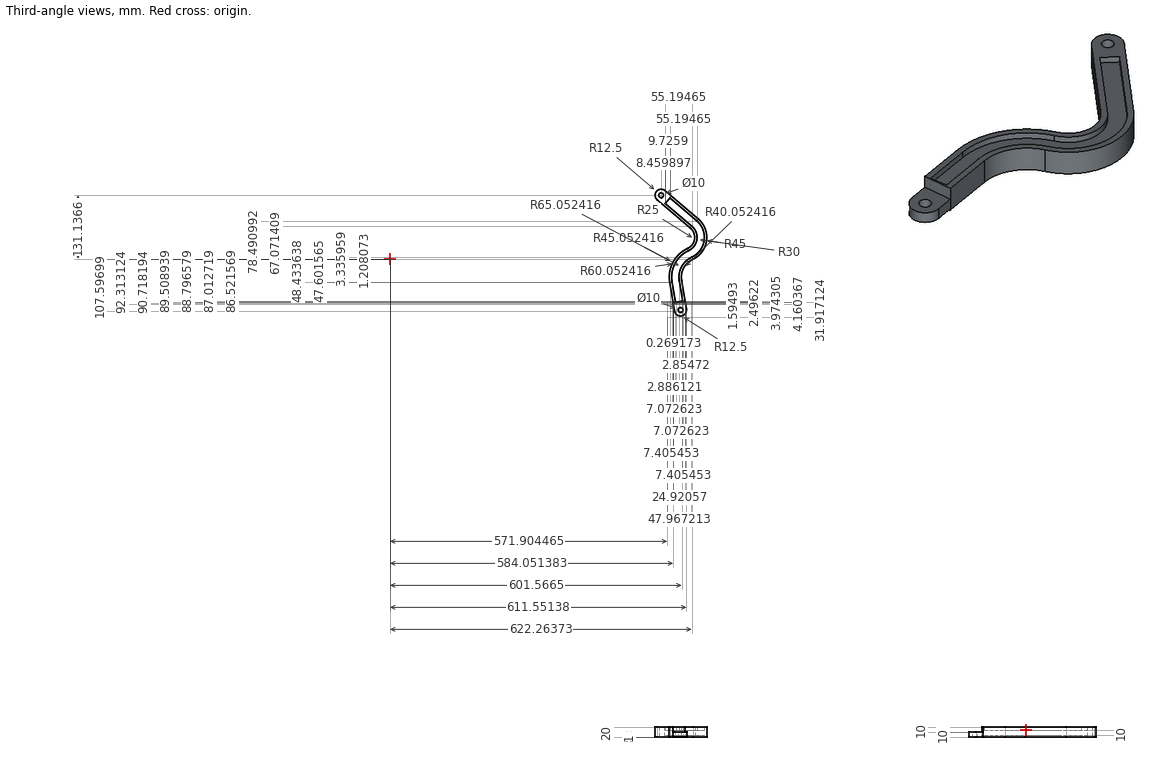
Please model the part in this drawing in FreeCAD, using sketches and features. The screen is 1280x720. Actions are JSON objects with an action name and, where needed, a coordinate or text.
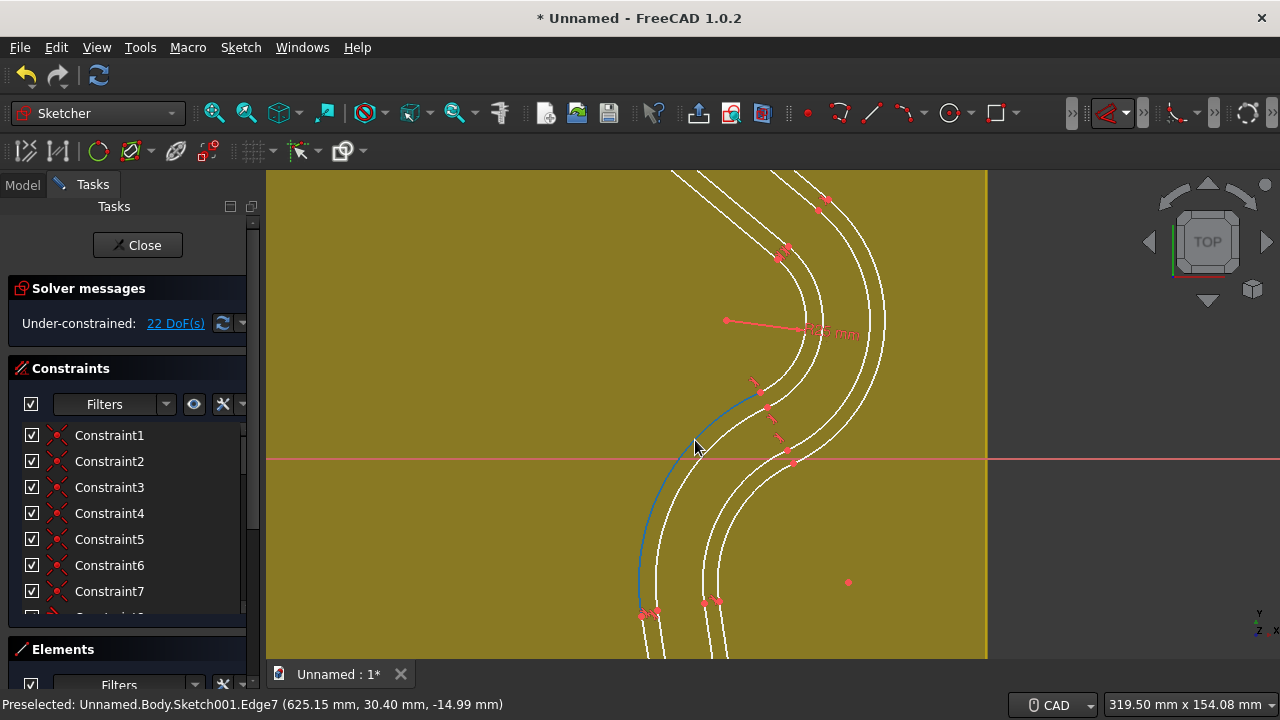
{"action": "left_click", "coordinate": [695, 440]}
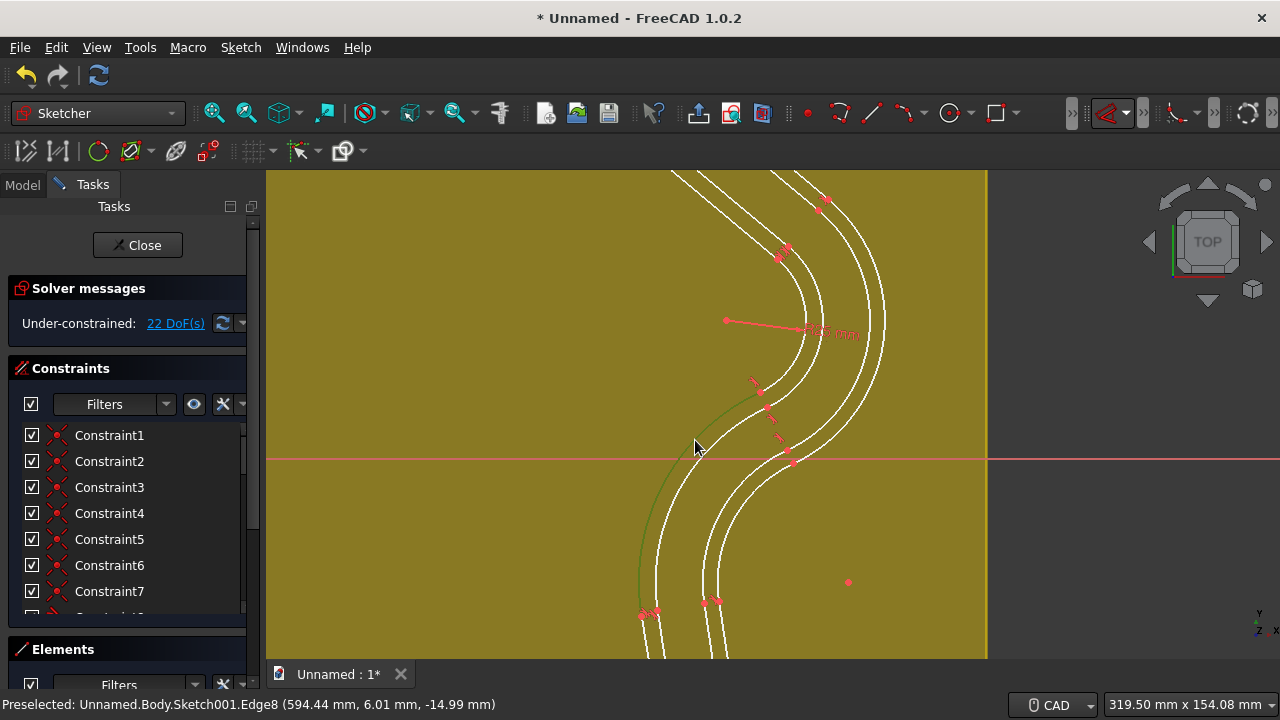
{"action": "key", "text": "k r"}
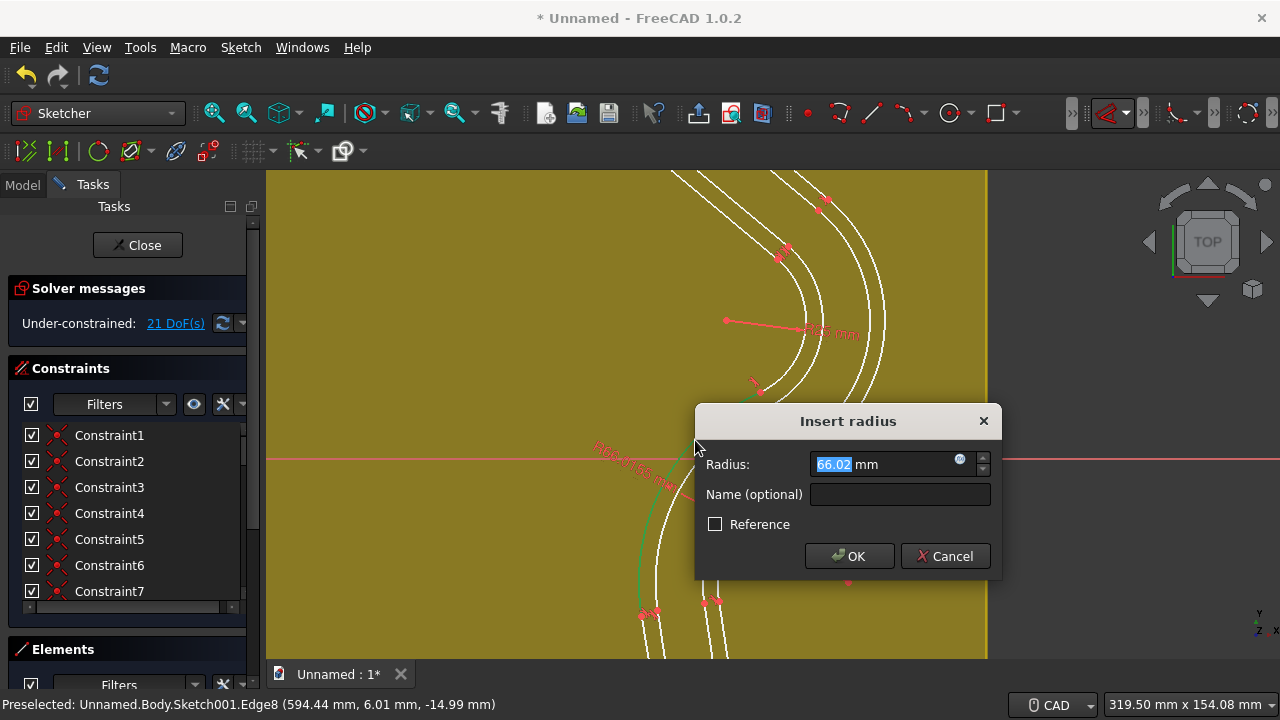
{"action": "type", "text": "65.052416"}
{"action": "key", "text": "Return"}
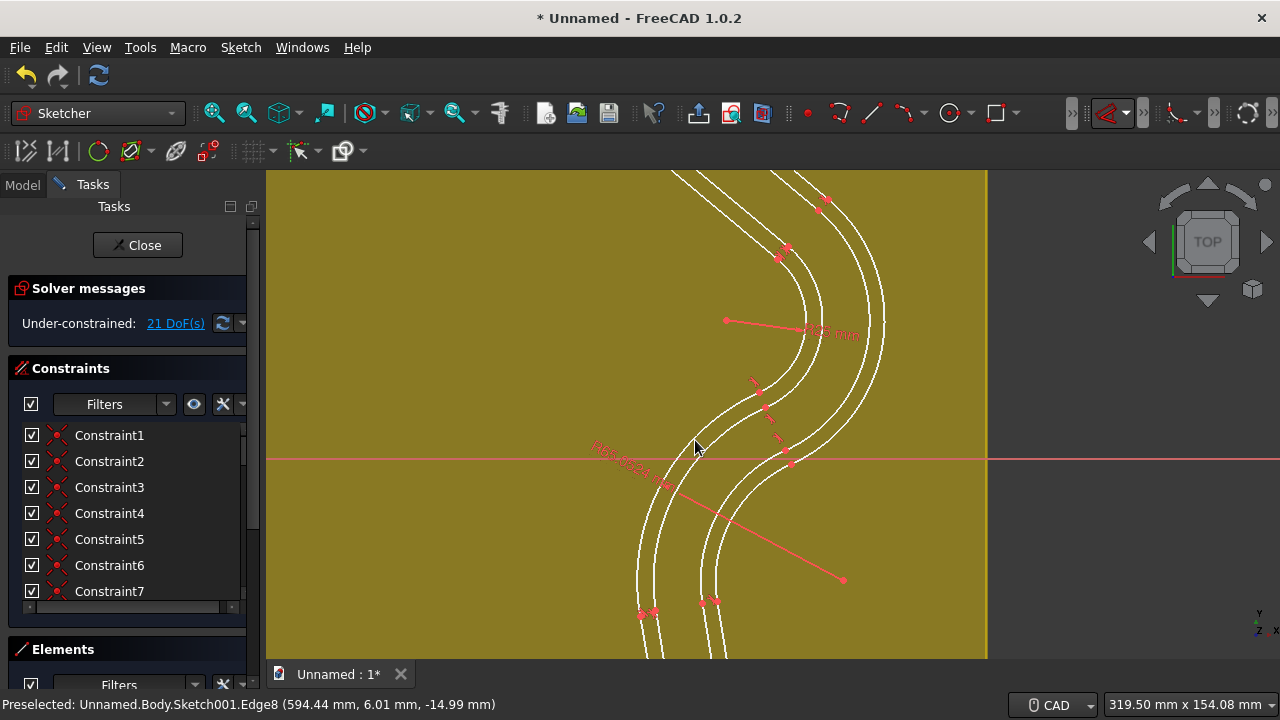
{"action": "left_click", "coordinate": [751, 493]}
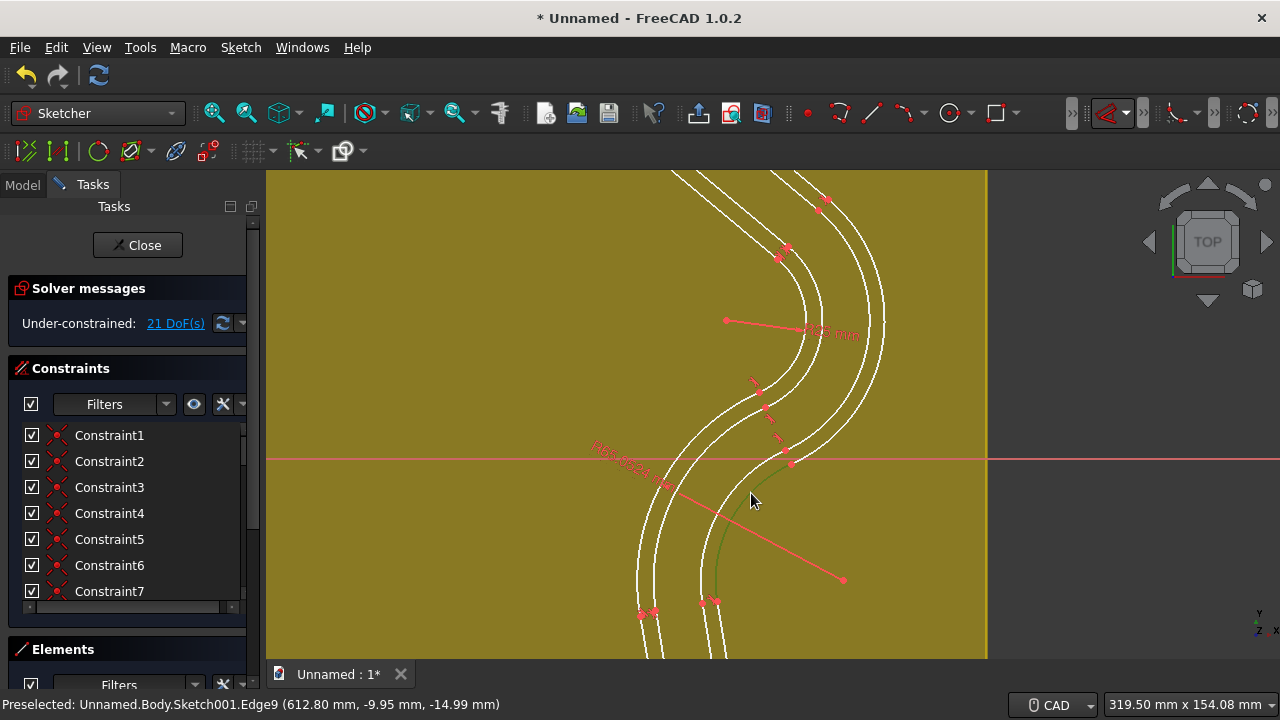
{"action": "left_click", "coordinate": [1128, 114]}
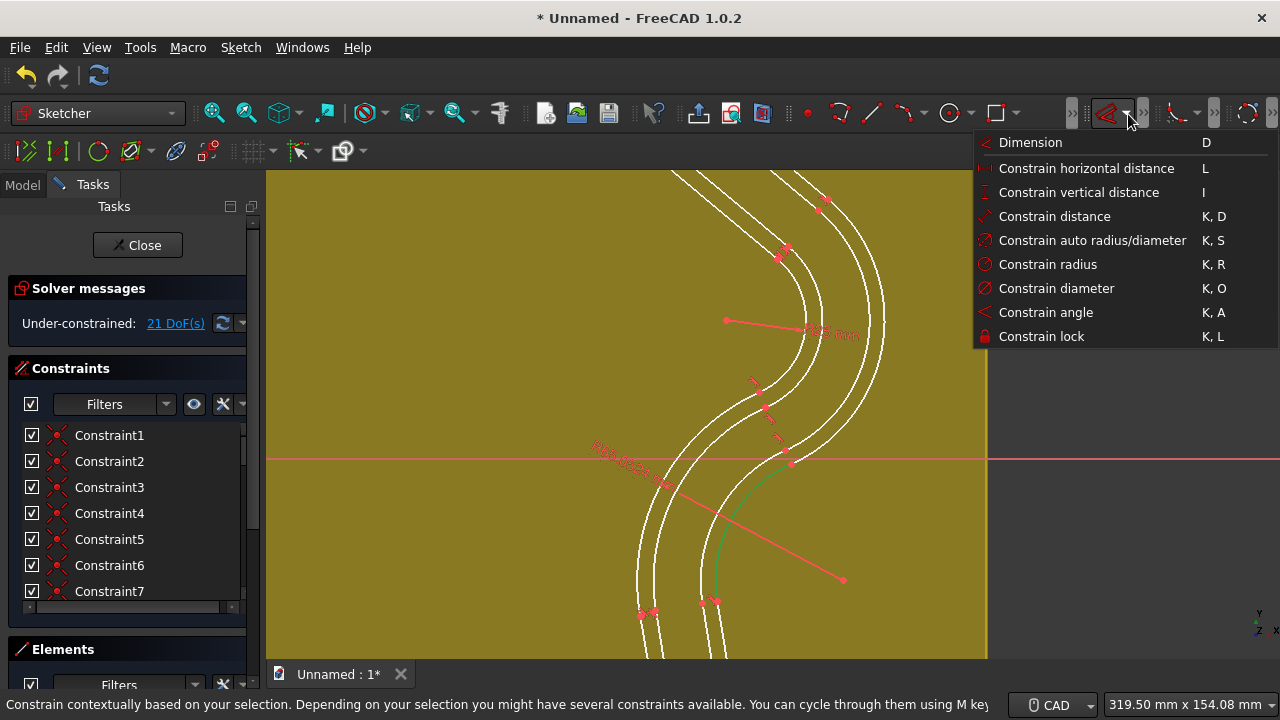
{"action": "left_click", "coordinate": [1126, 264]}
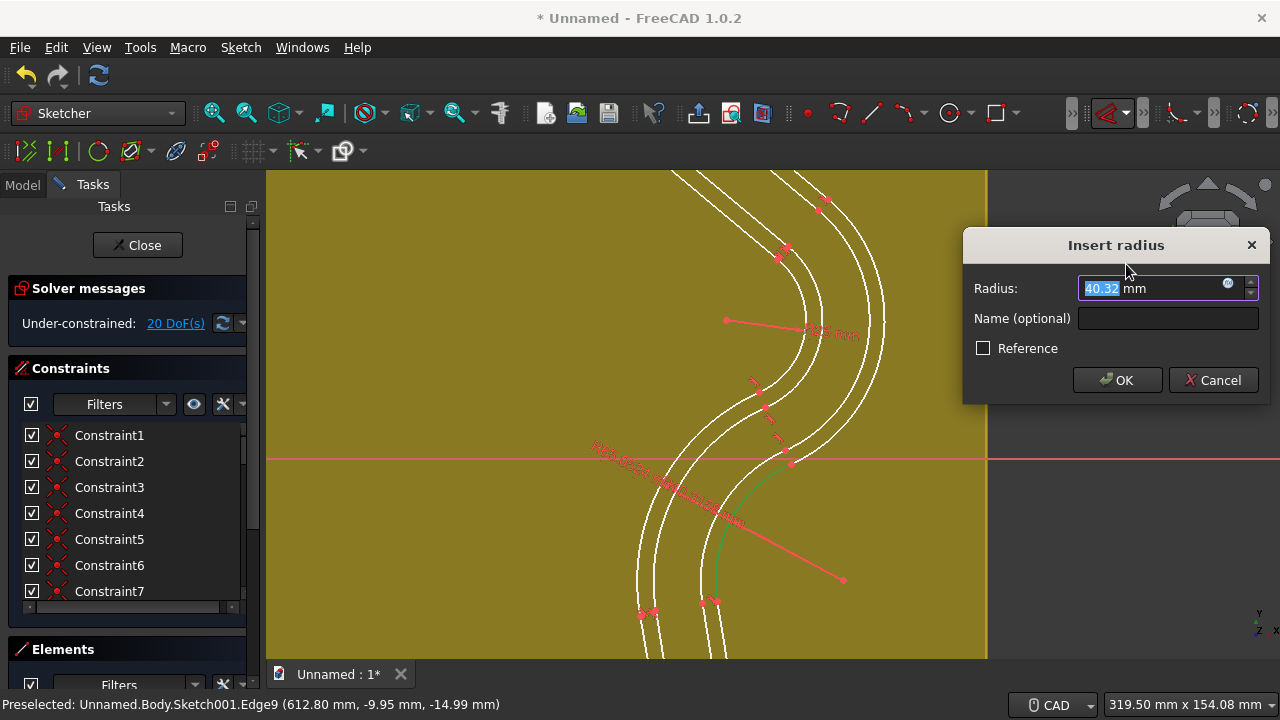
{"action": "type", "text": "40.052416"}
{"action": "key", "text": "Return"}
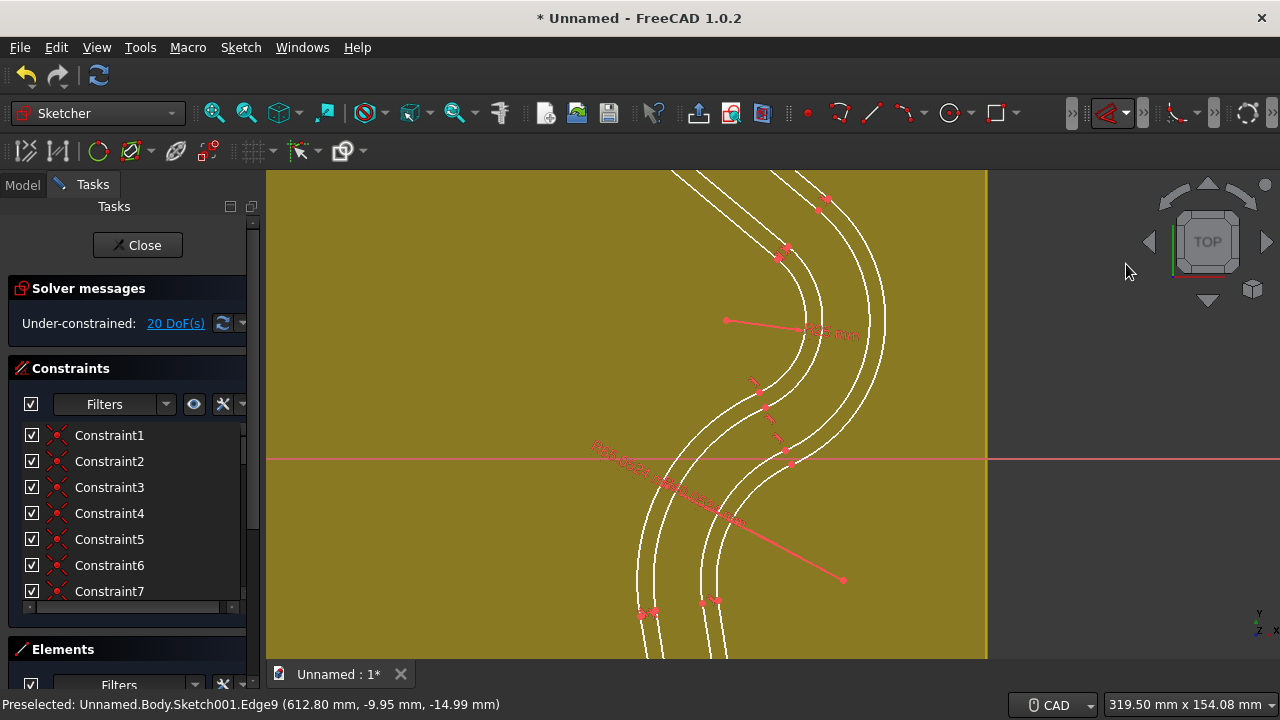
{"action": "left_click", "coordinate": [659, 537]}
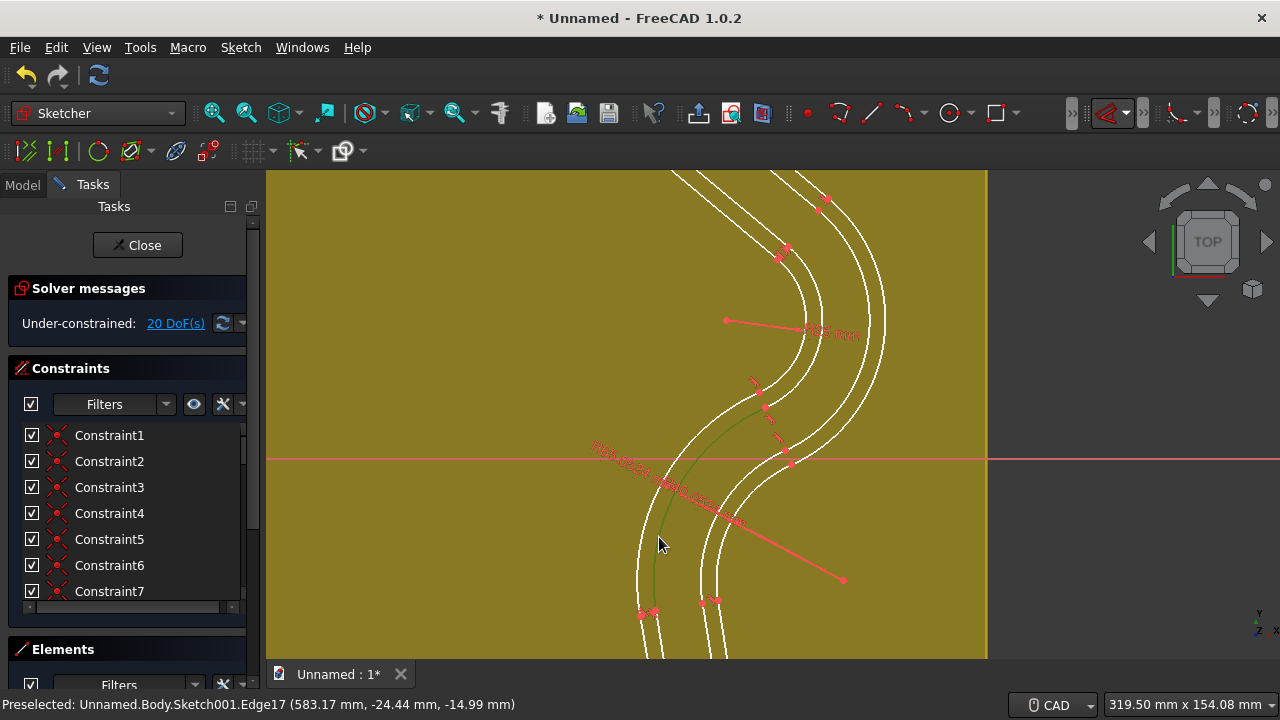
{"action": "left_click", "coordinate": [1128, 114]}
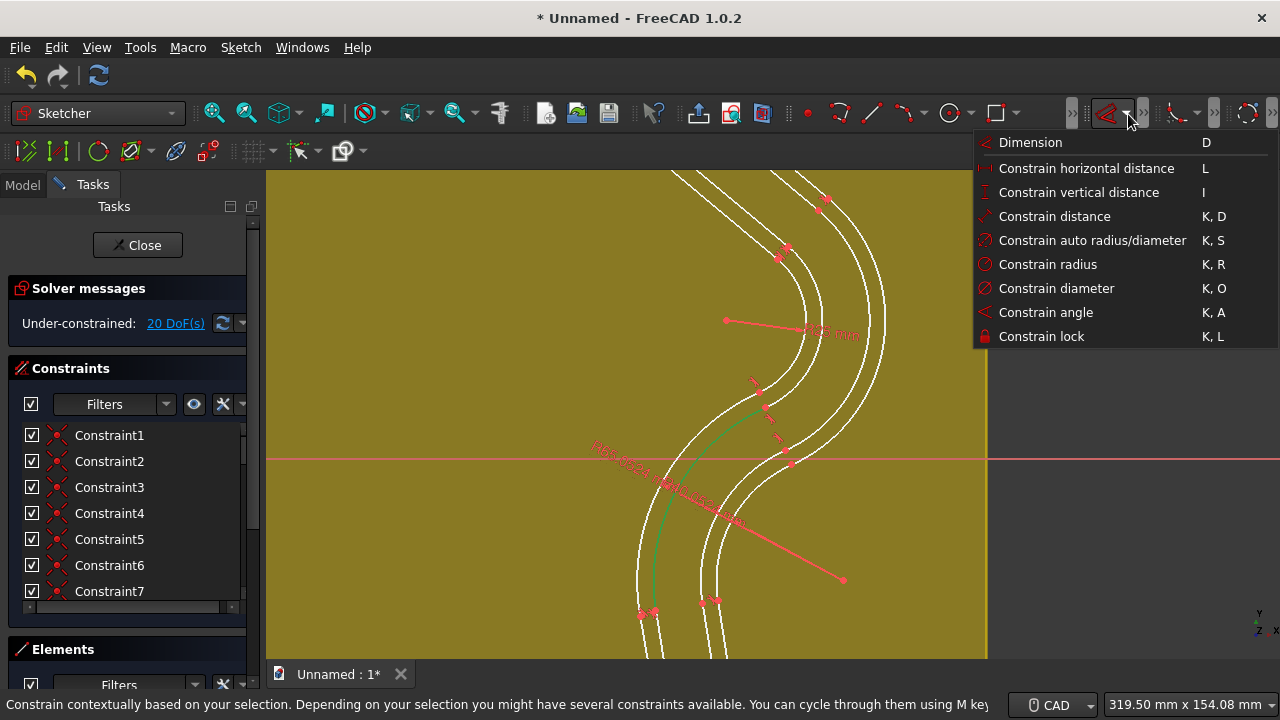
{"action": "left_click", "coordinate": [1126, 264]}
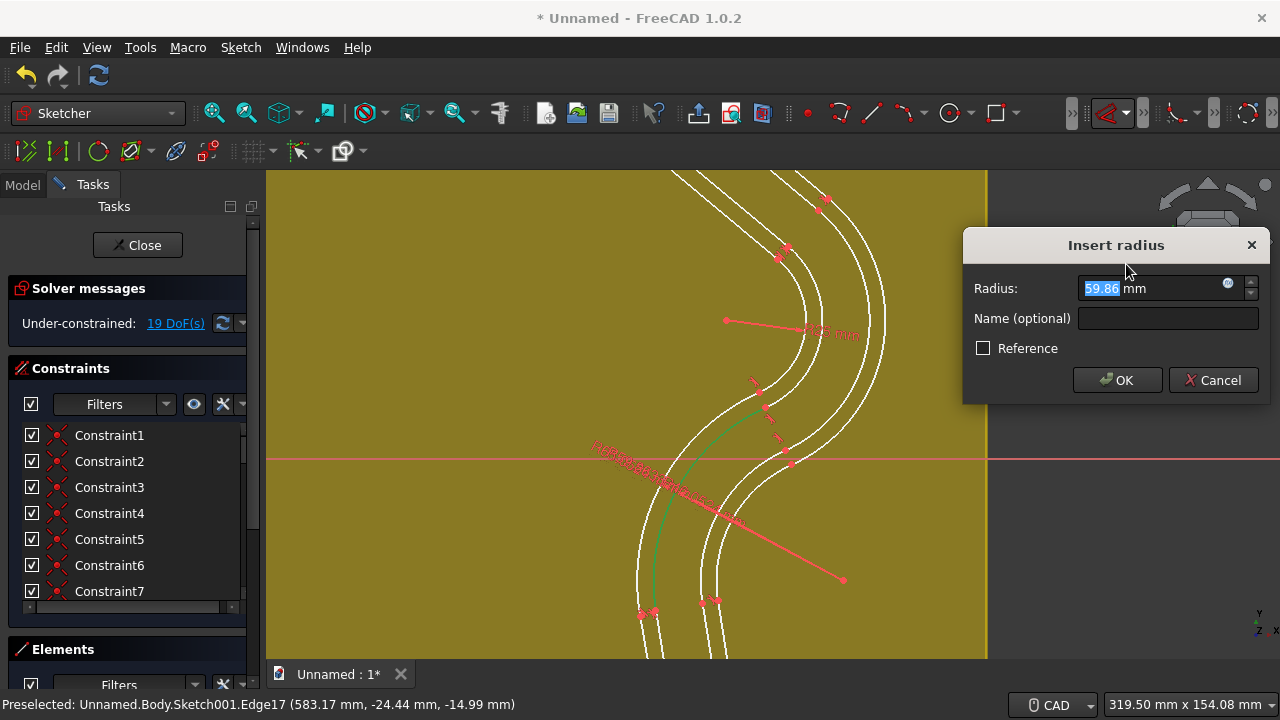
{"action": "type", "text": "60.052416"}
{"action": "key", "text": "Return"}